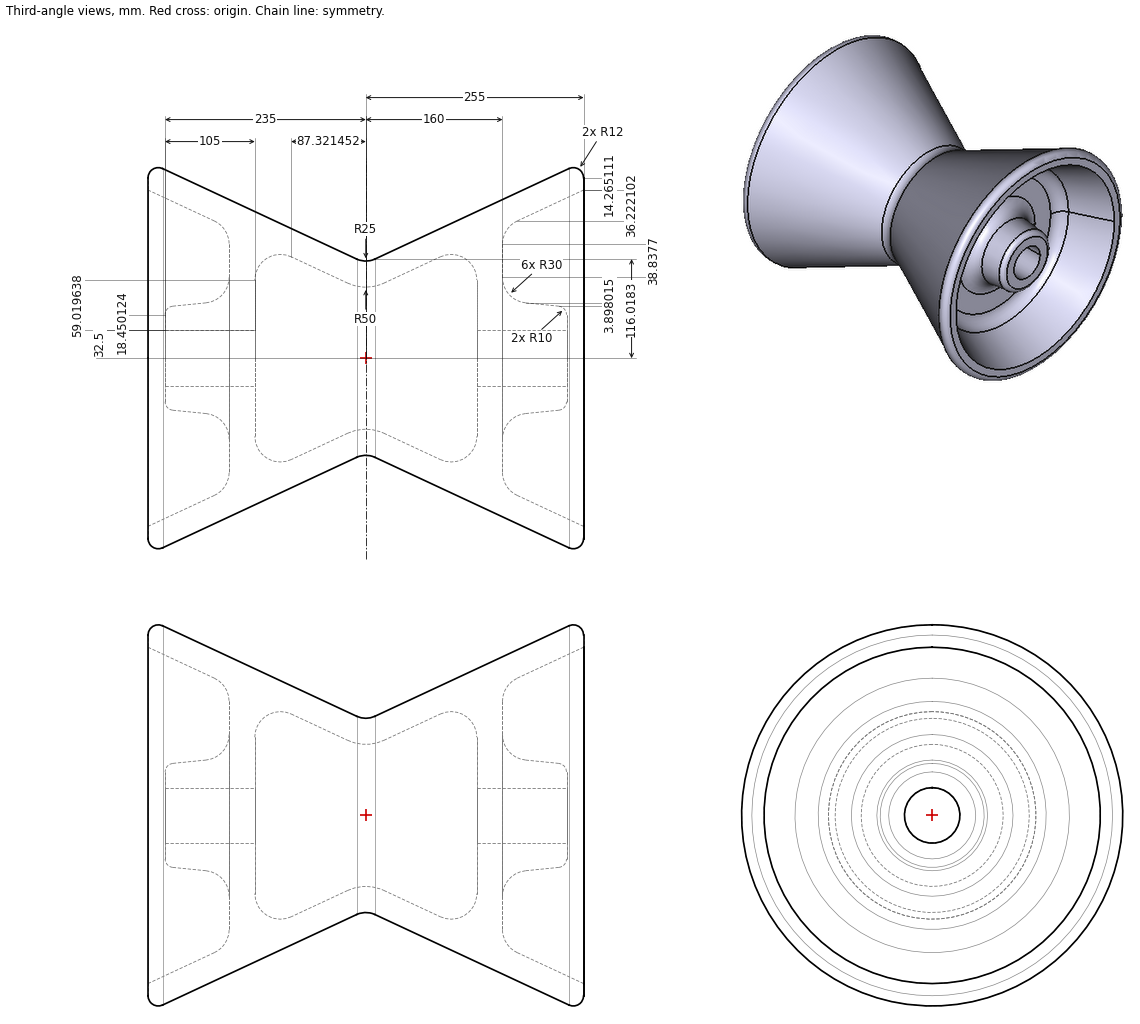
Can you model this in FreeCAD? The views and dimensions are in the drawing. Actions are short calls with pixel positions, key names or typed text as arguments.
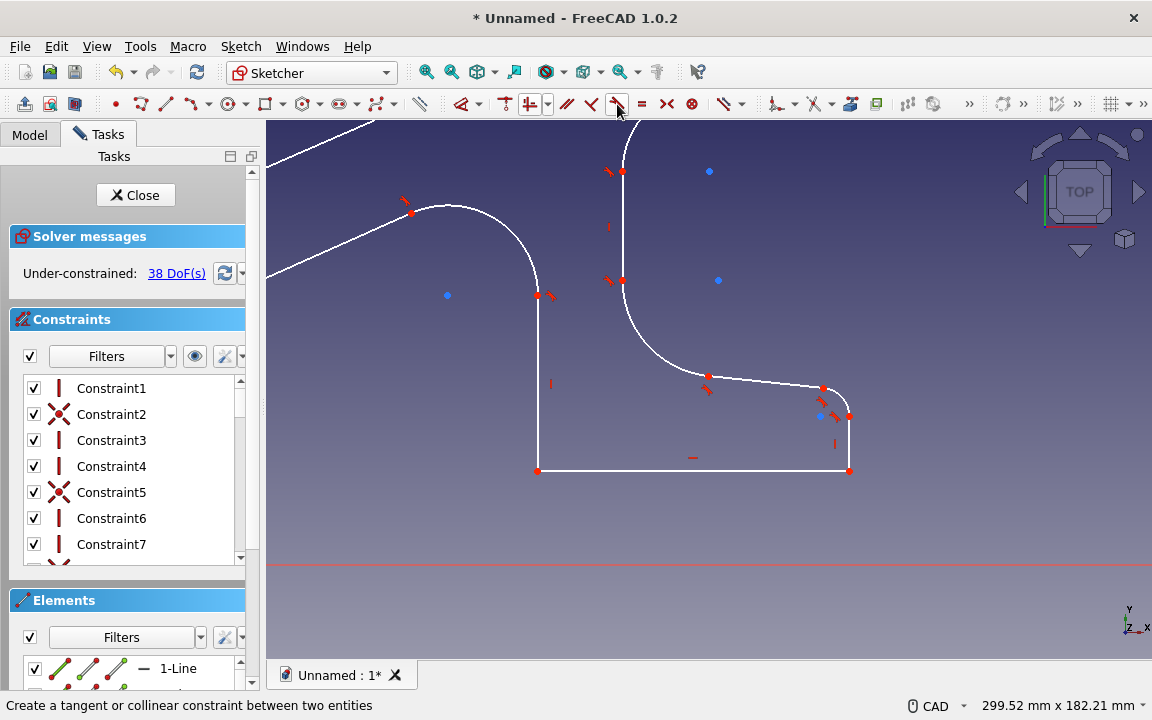
click(632, 322)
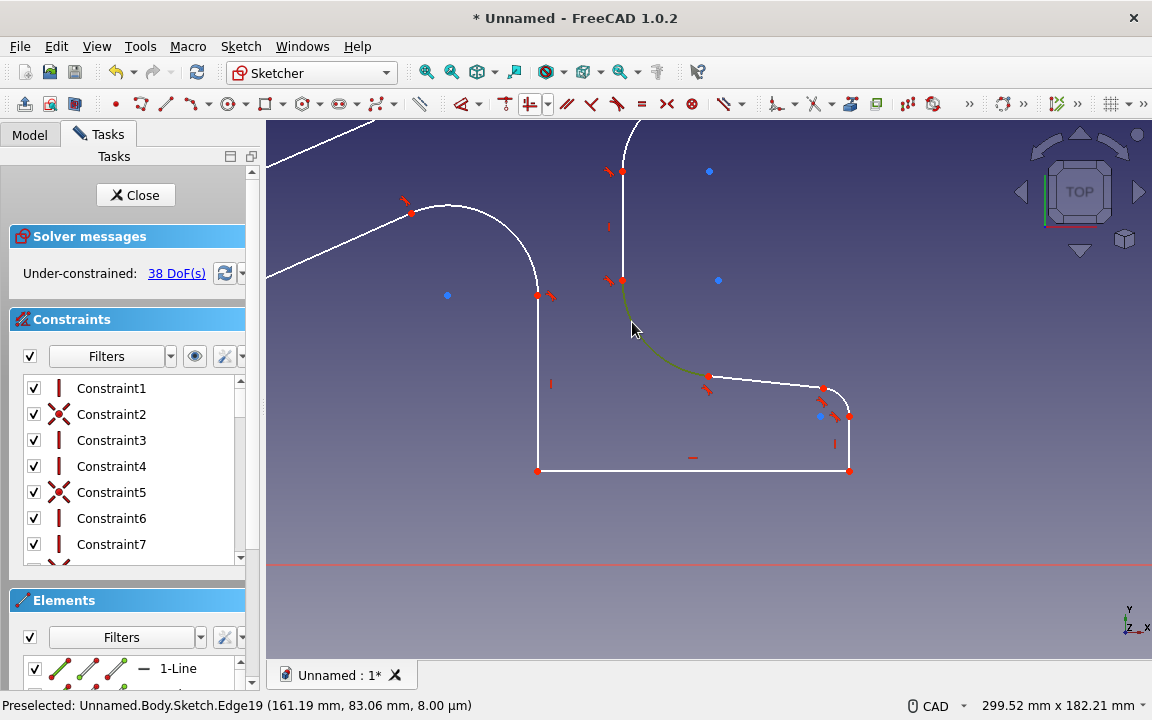
click(625, 152)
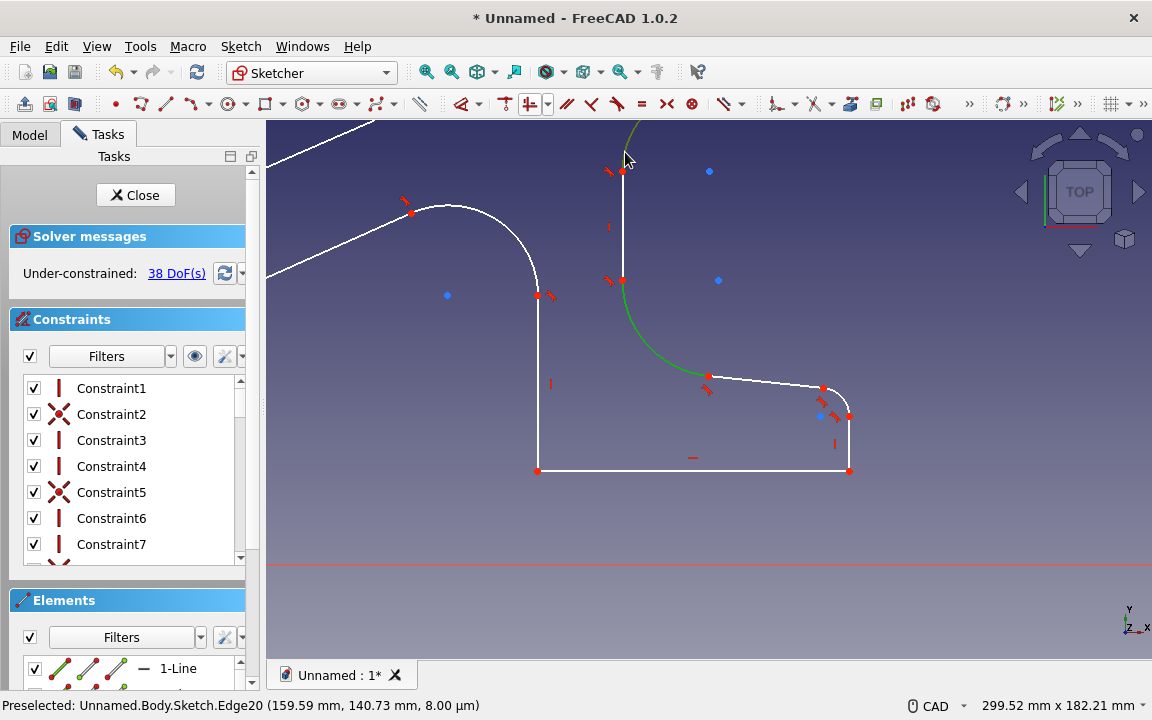
scroll(850, 456, down, 6)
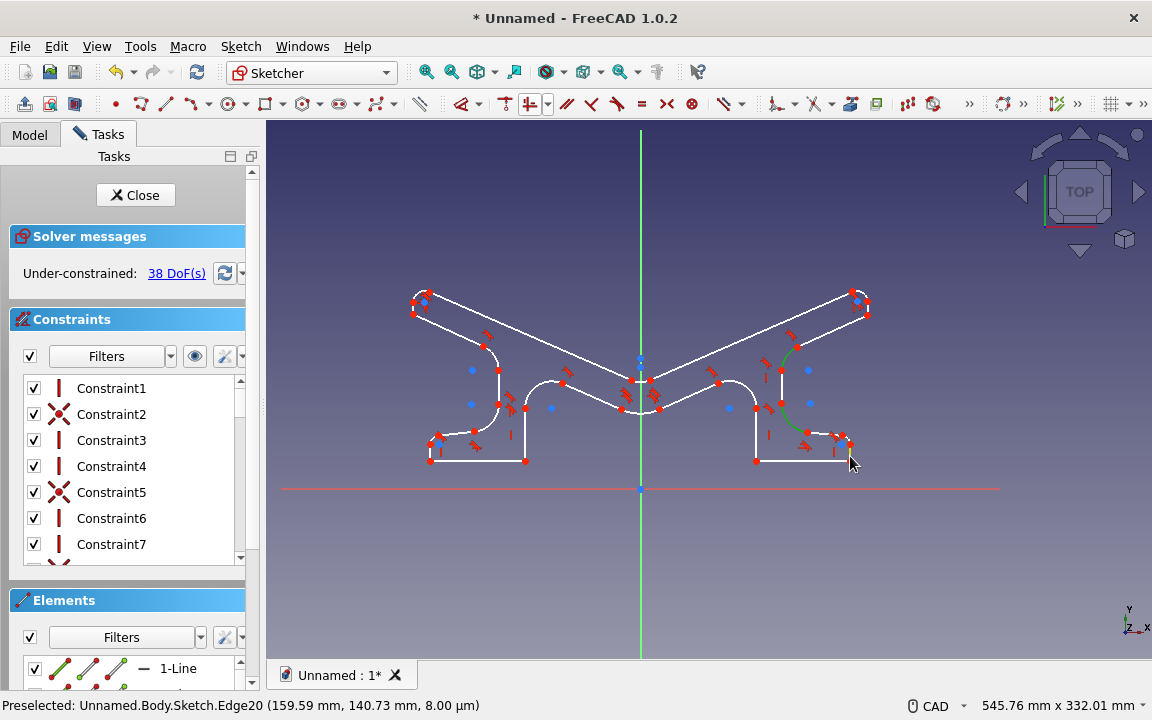
scroll(497, 362, up, 3)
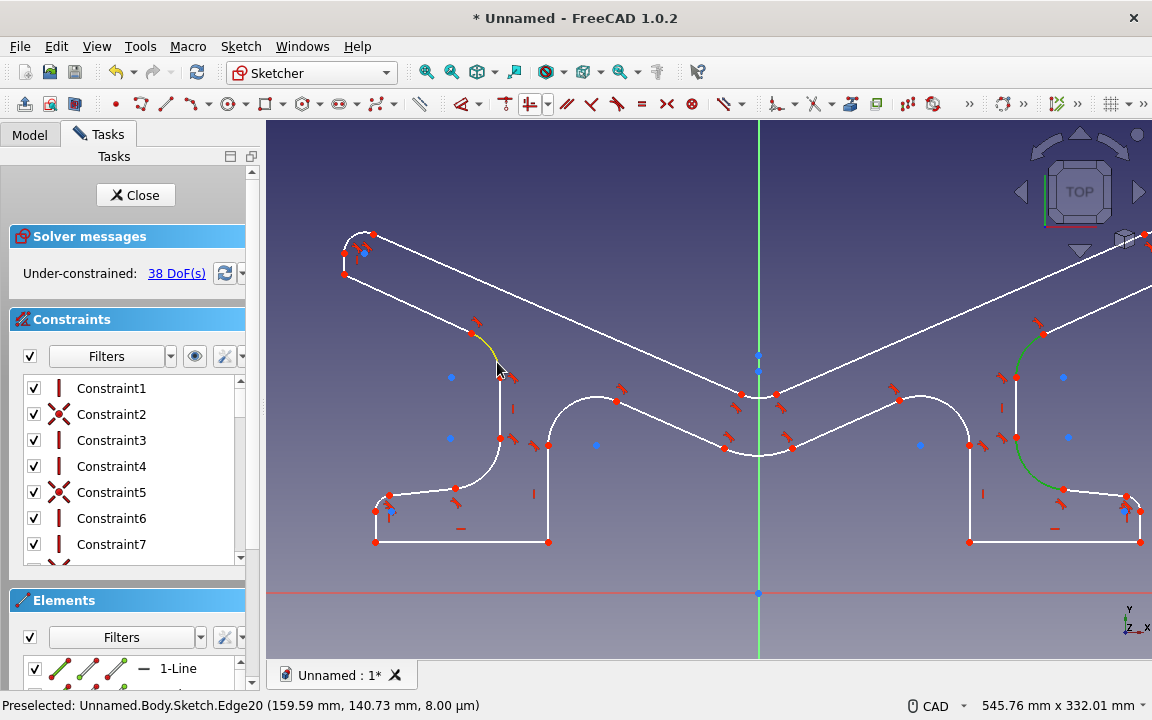
click(497, 361)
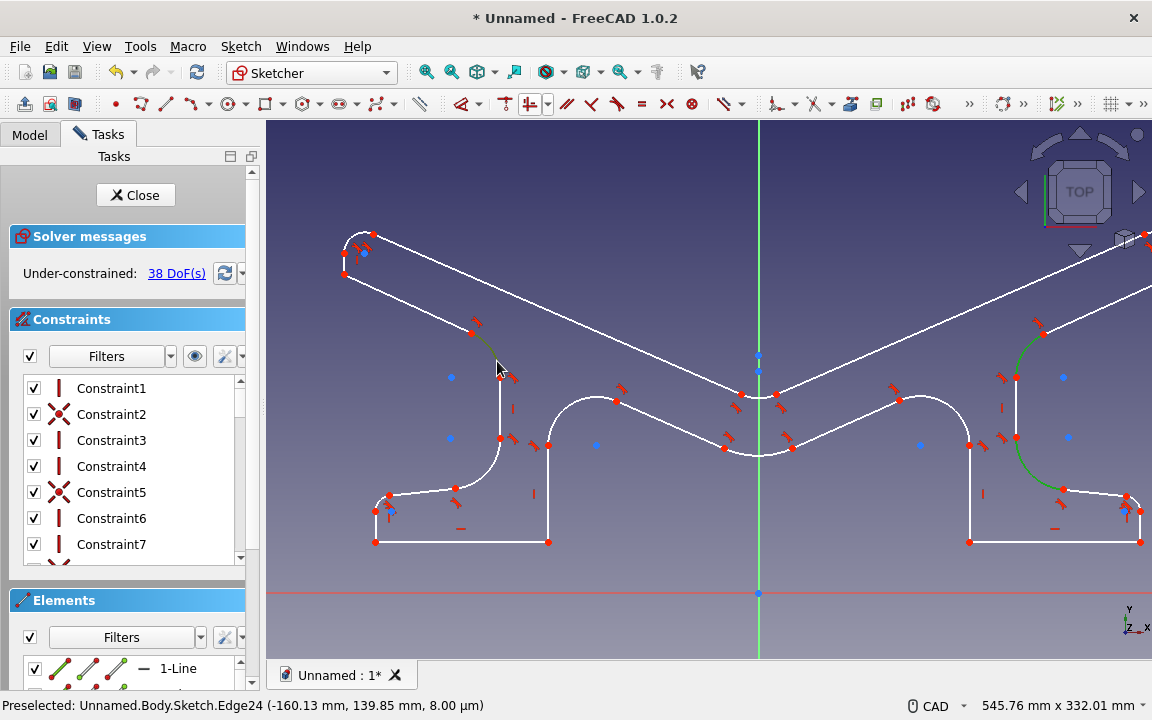
click(476, 482)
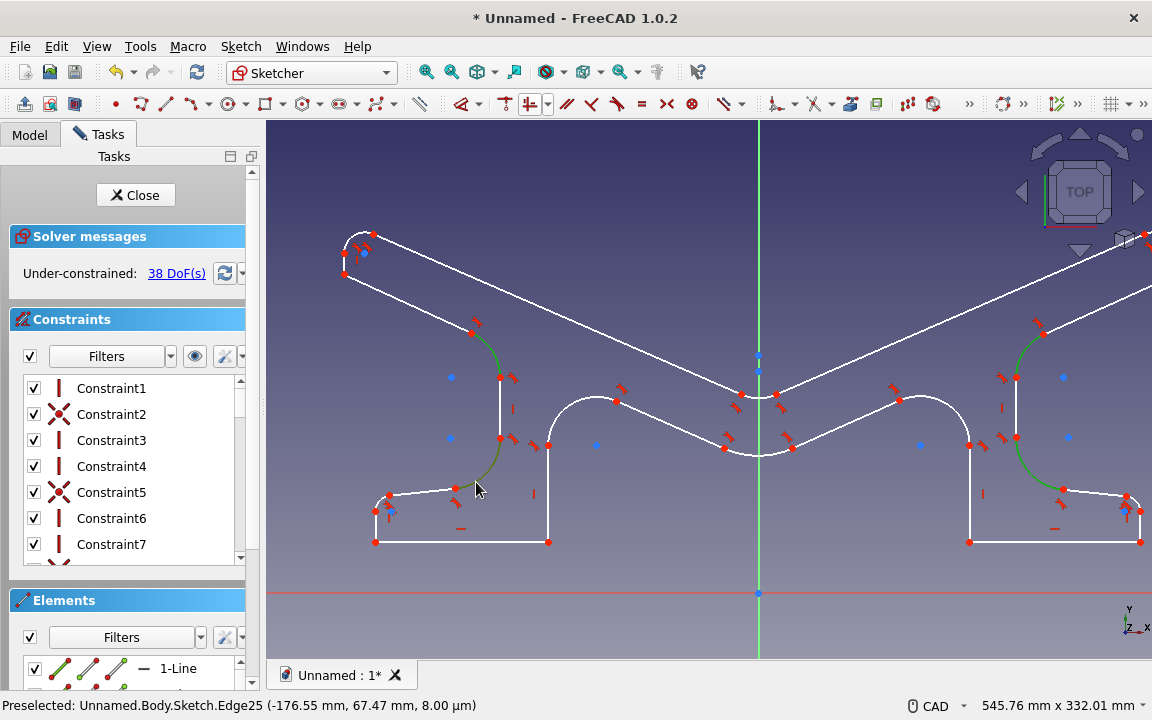
click(588, 398)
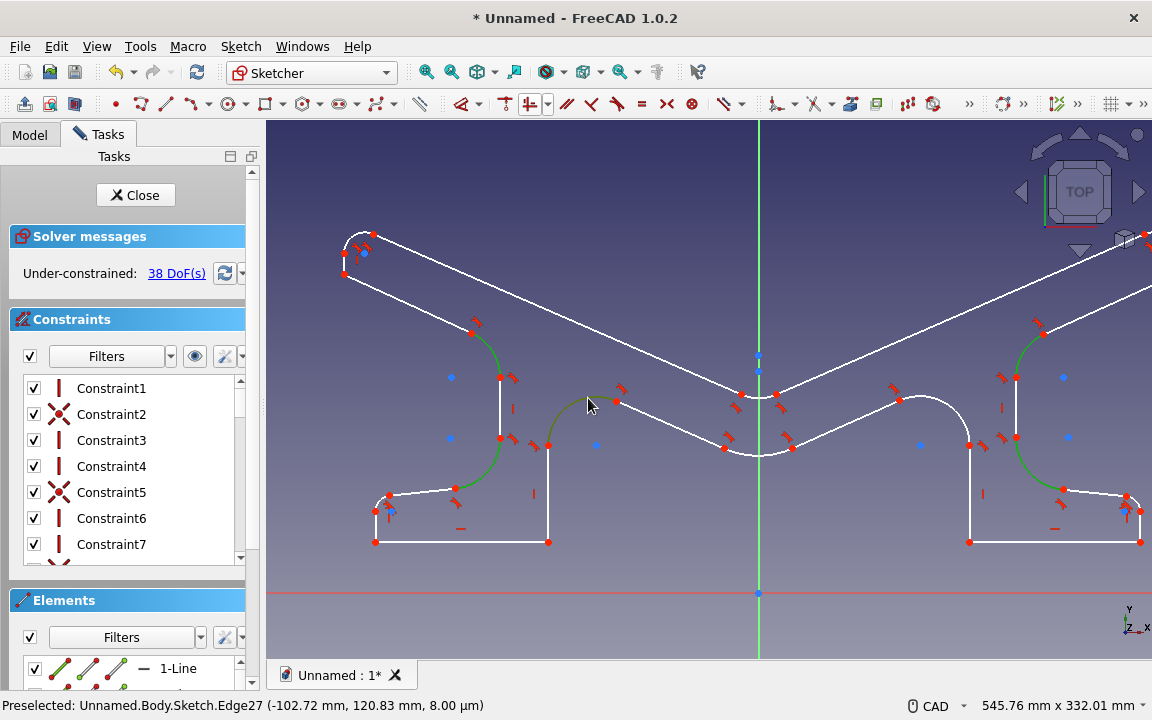
click(961, 418)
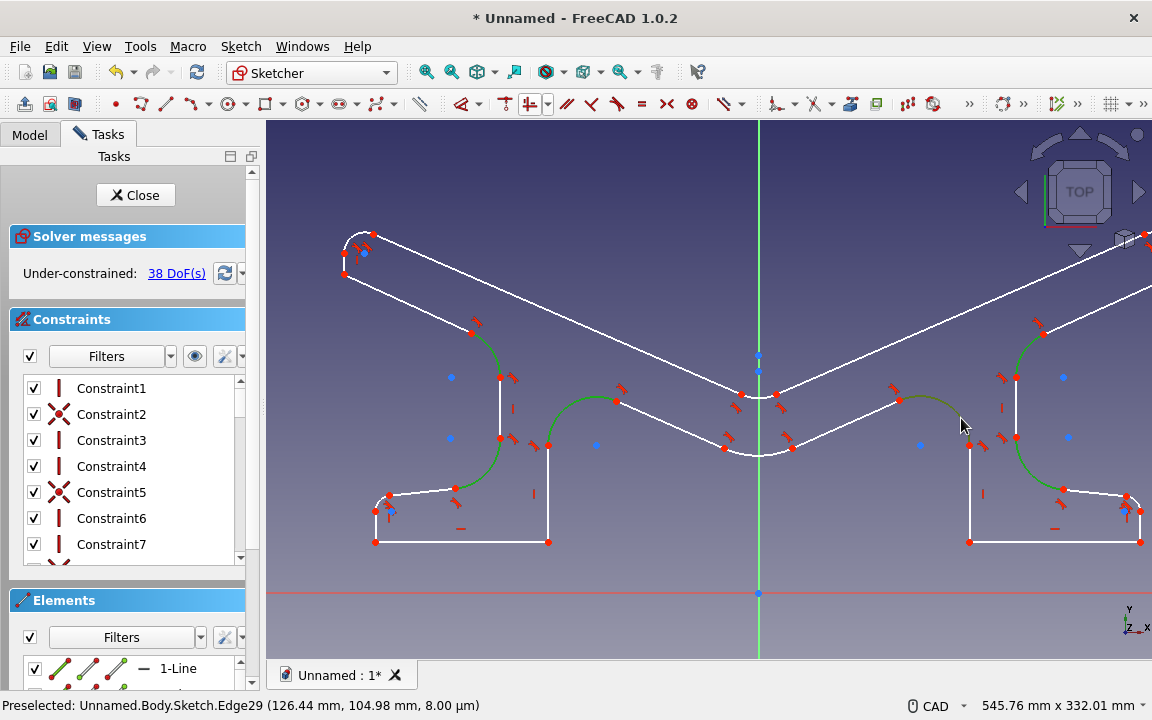
key(e)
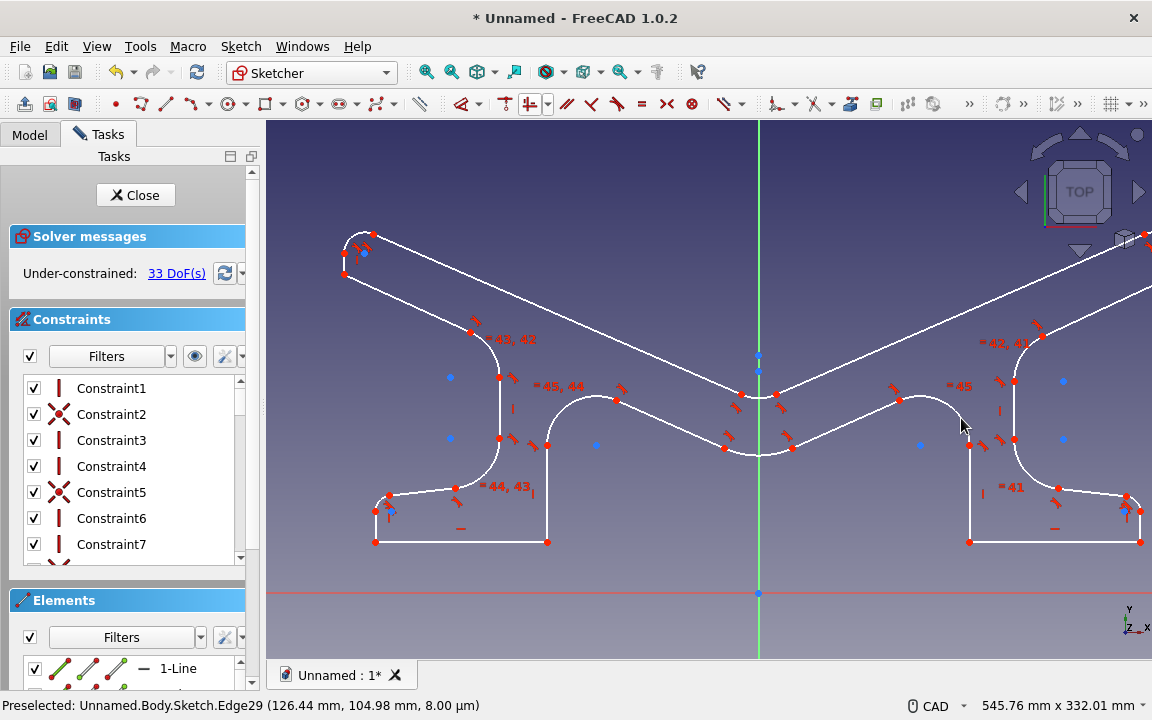
scroll(497, 361, down, 3)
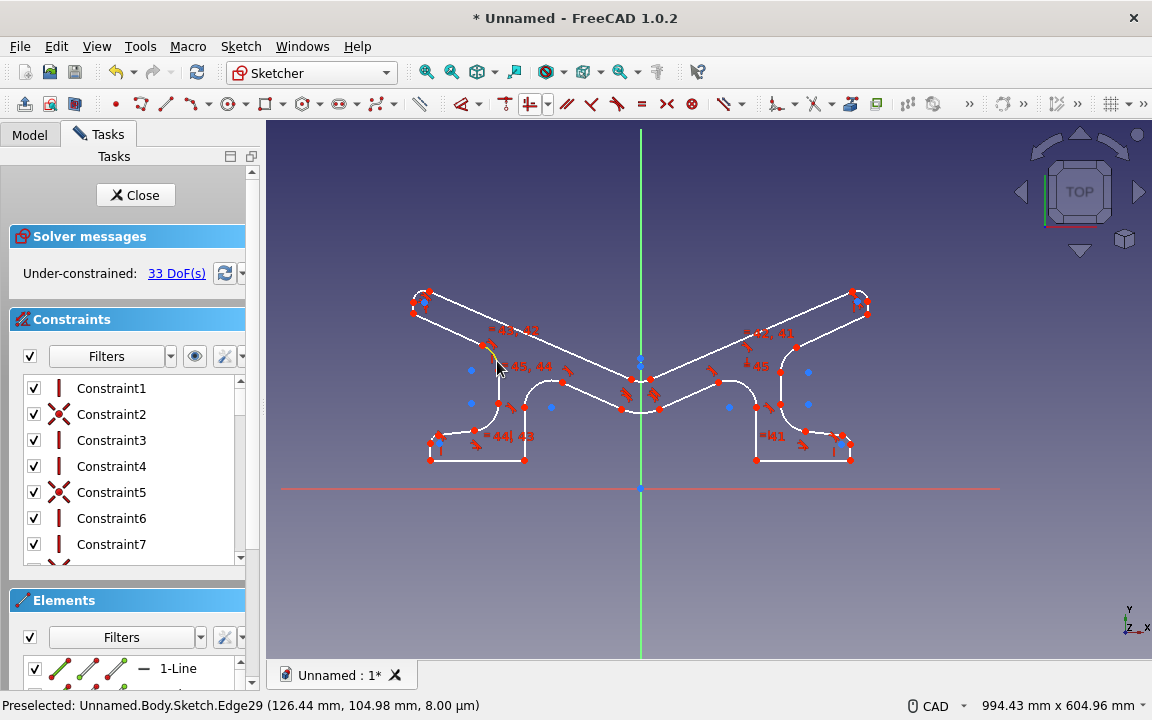
scroll(866, 295, up, 4)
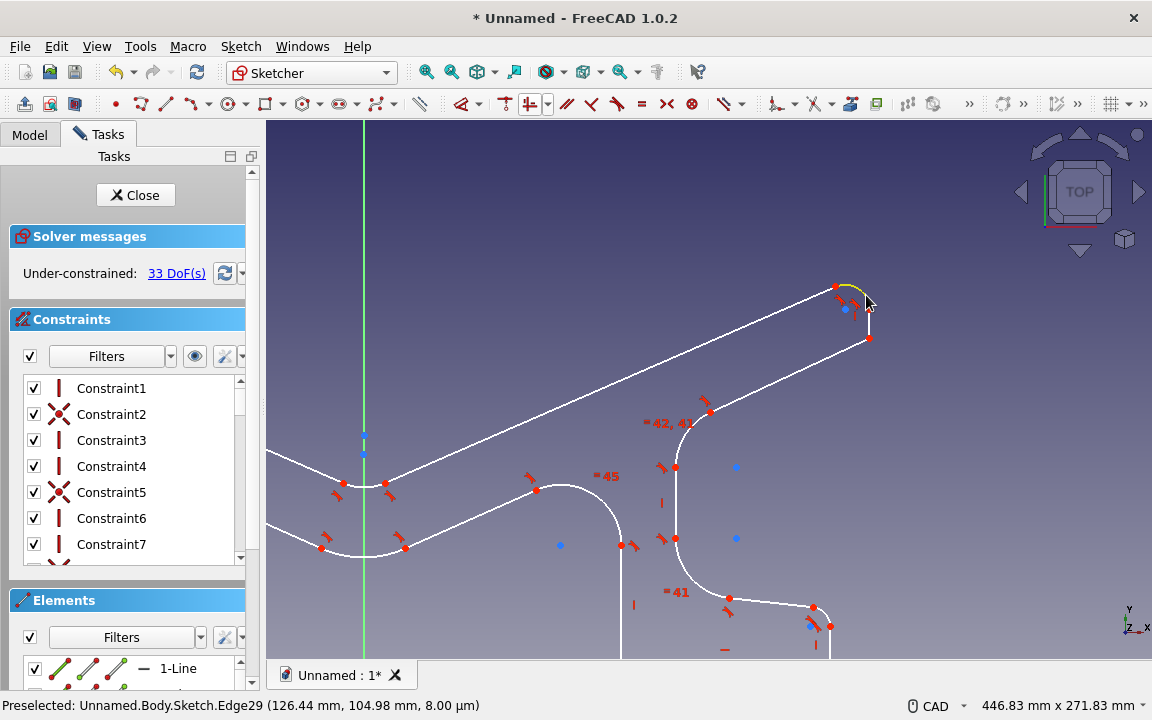
click(865, 295)